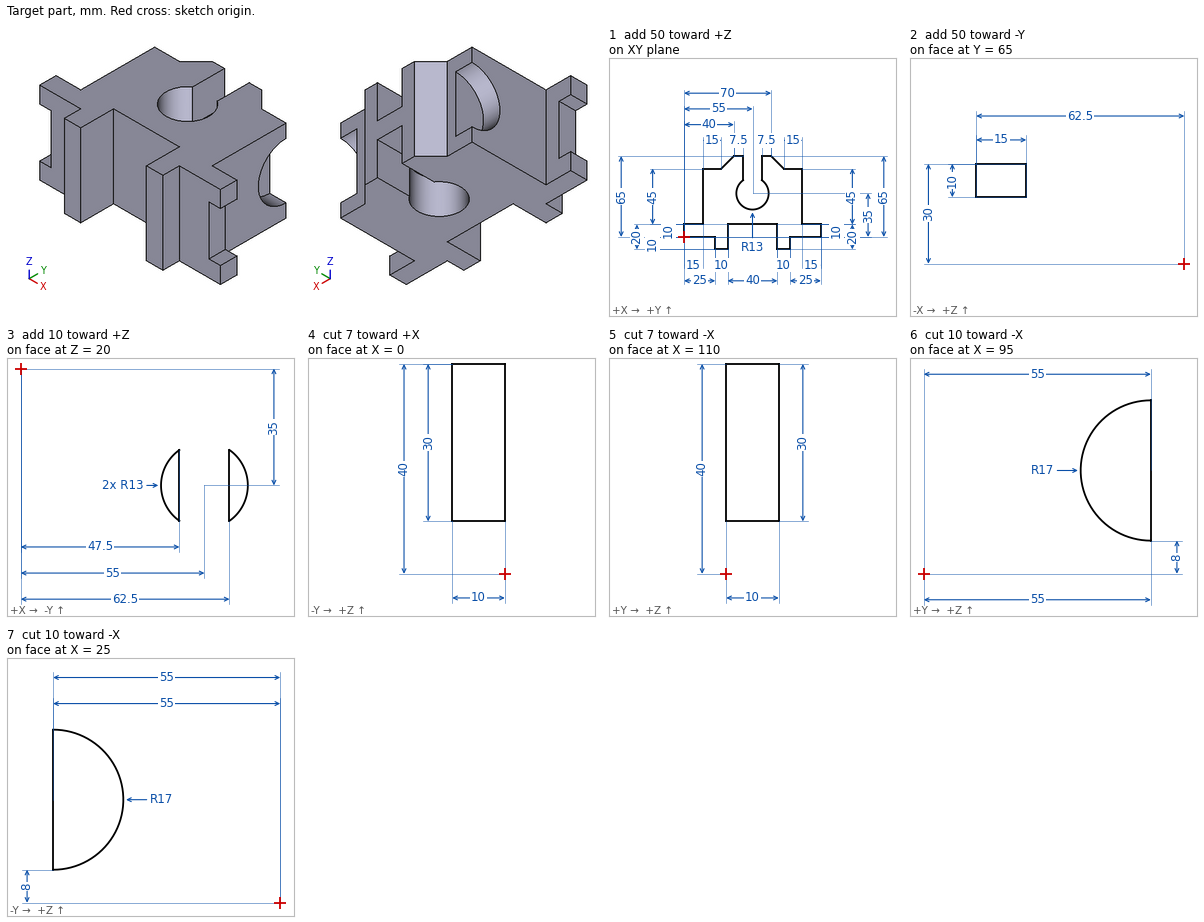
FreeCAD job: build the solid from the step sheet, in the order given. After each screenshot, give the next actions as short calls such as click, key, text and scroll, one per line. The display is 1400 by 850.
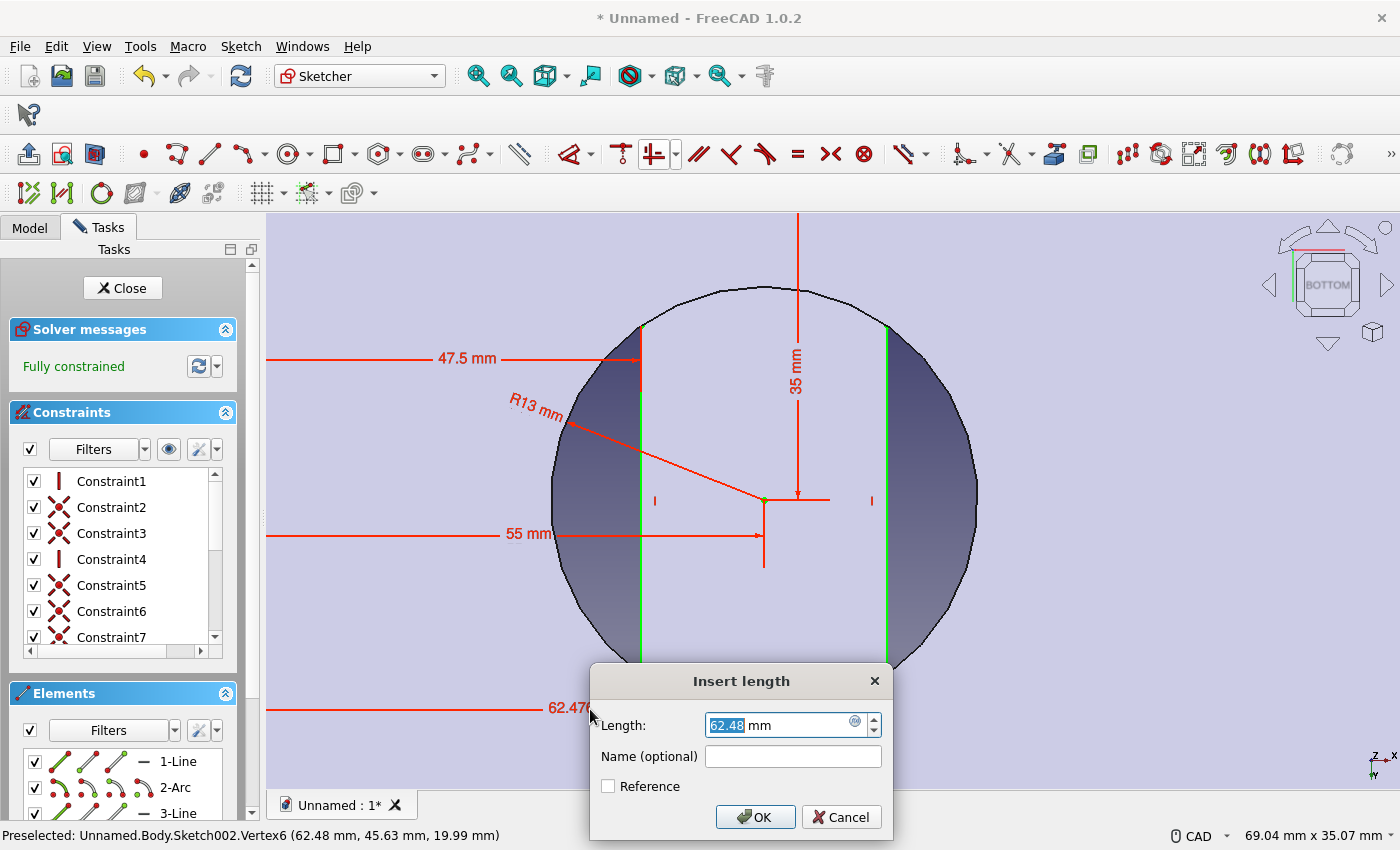
text(62.5)
key(Return)
key(Escape)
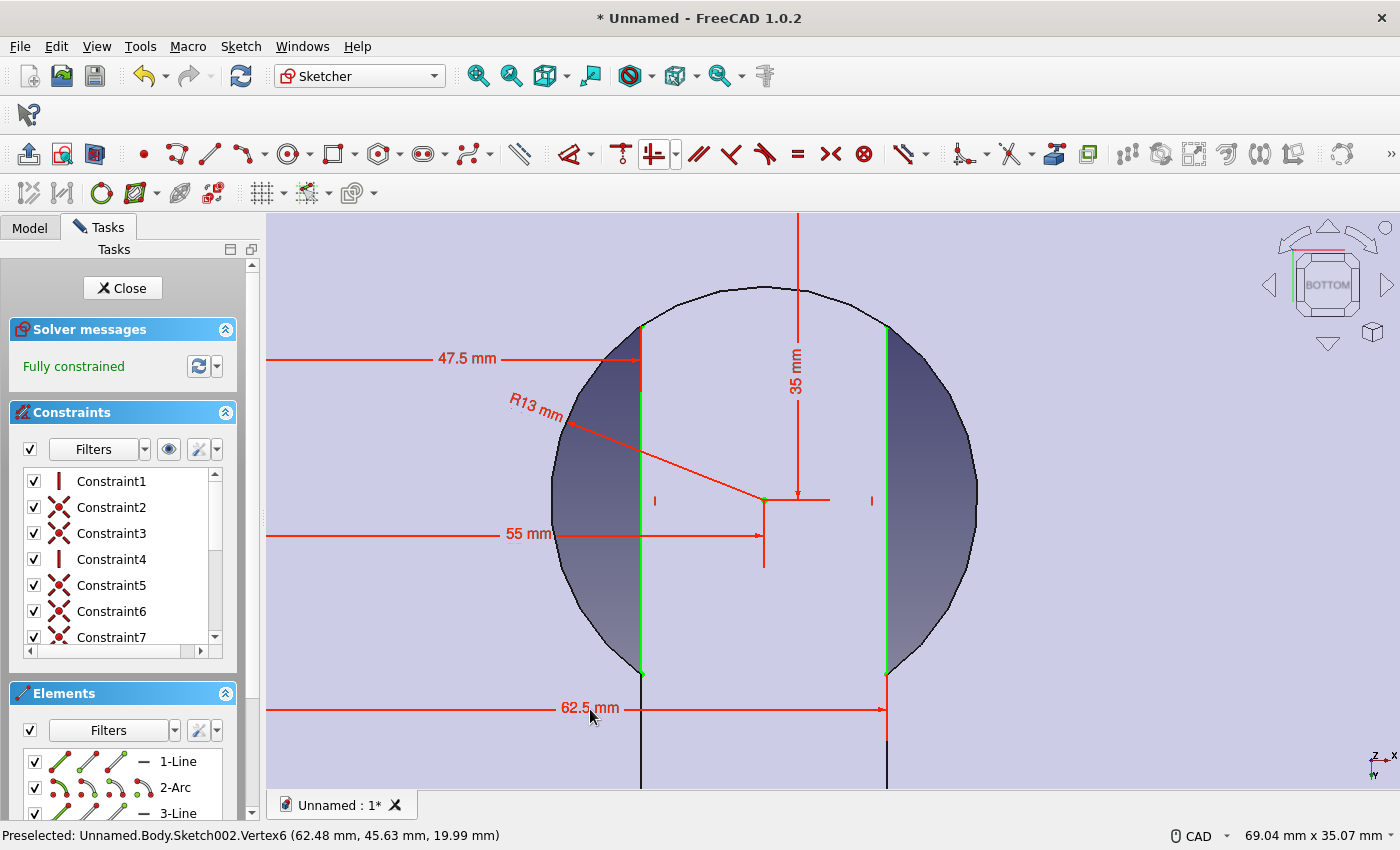
click(123, 288)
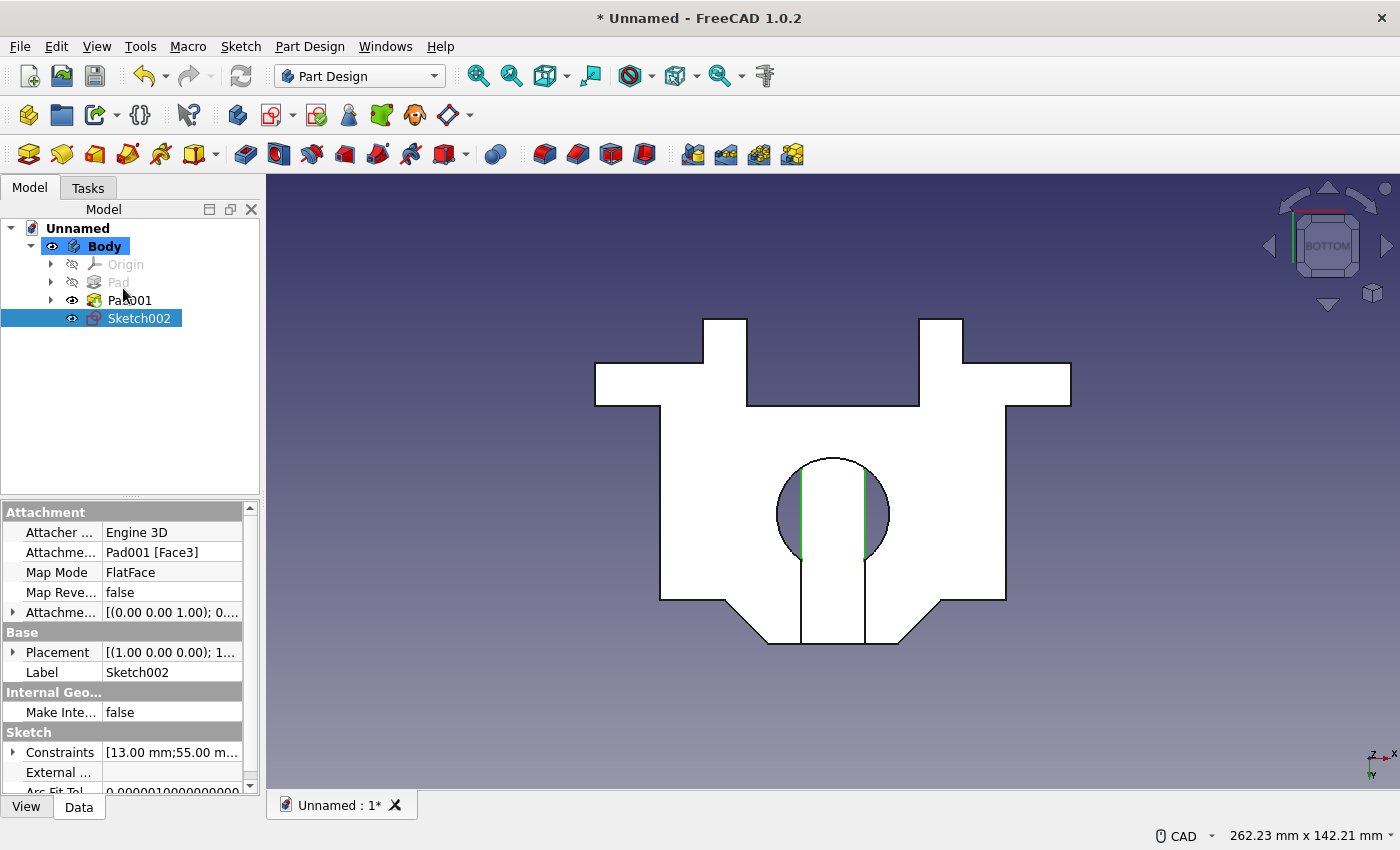
click(29, 154)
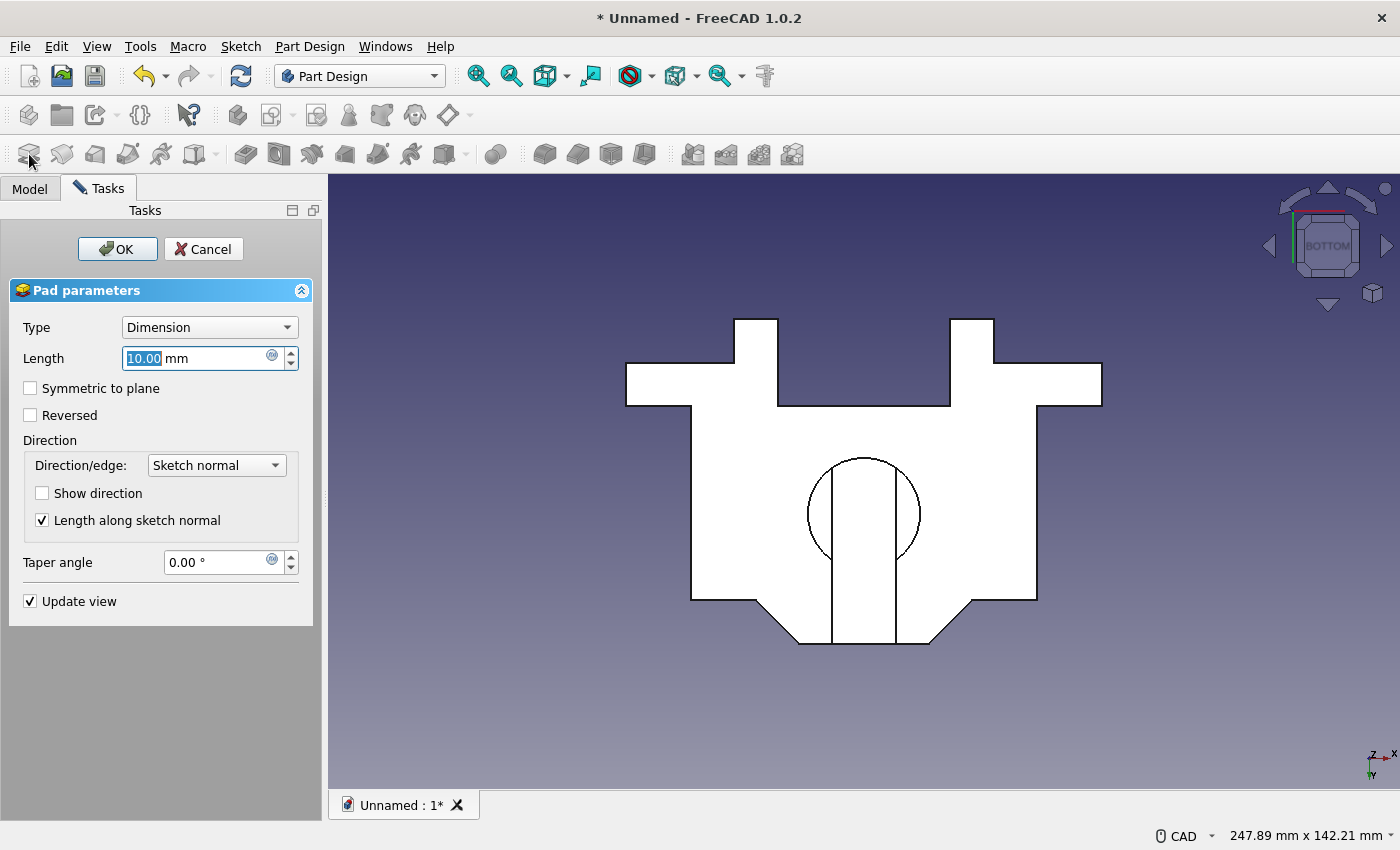
text(10)
key(Tab)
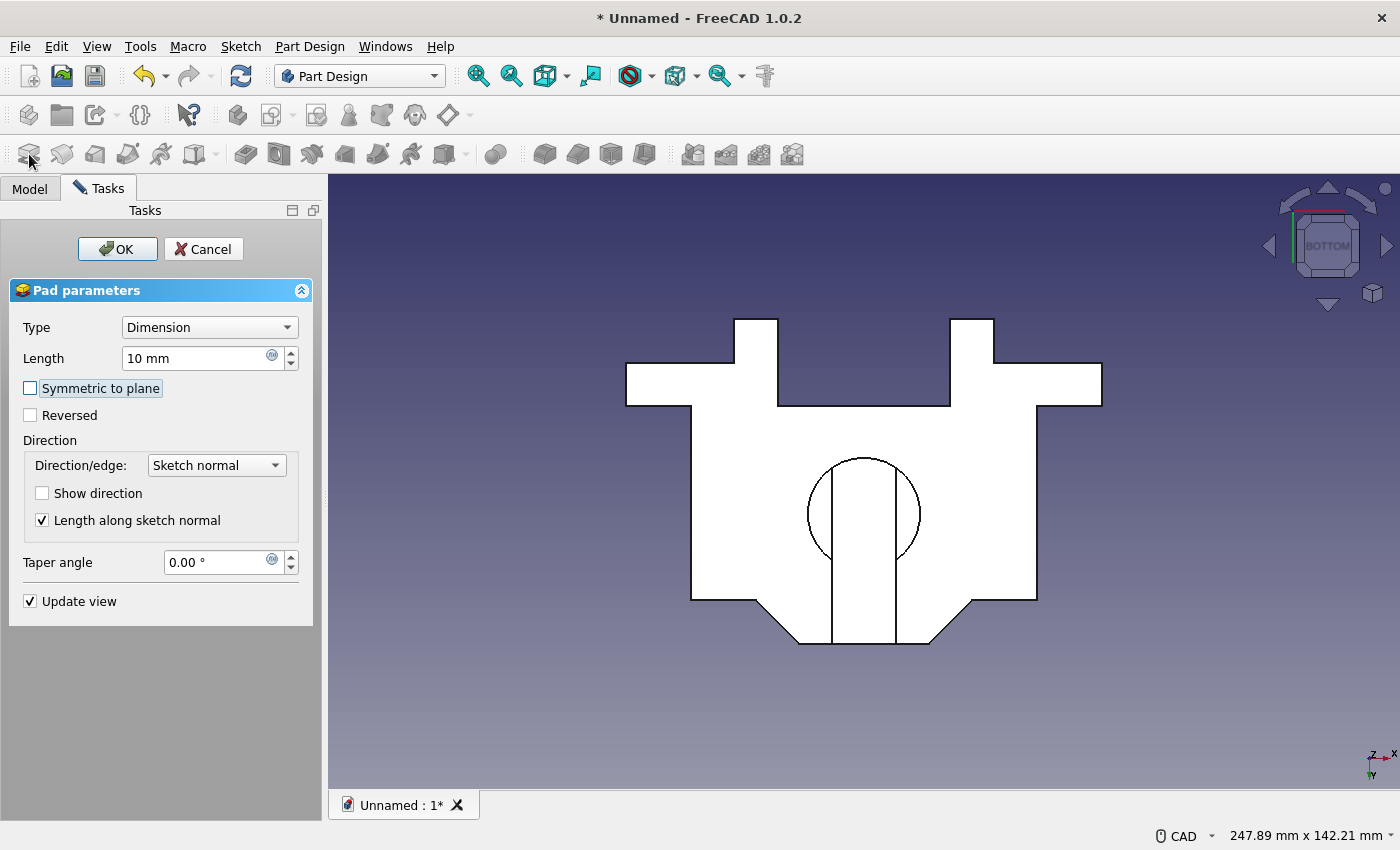
click(31, 415)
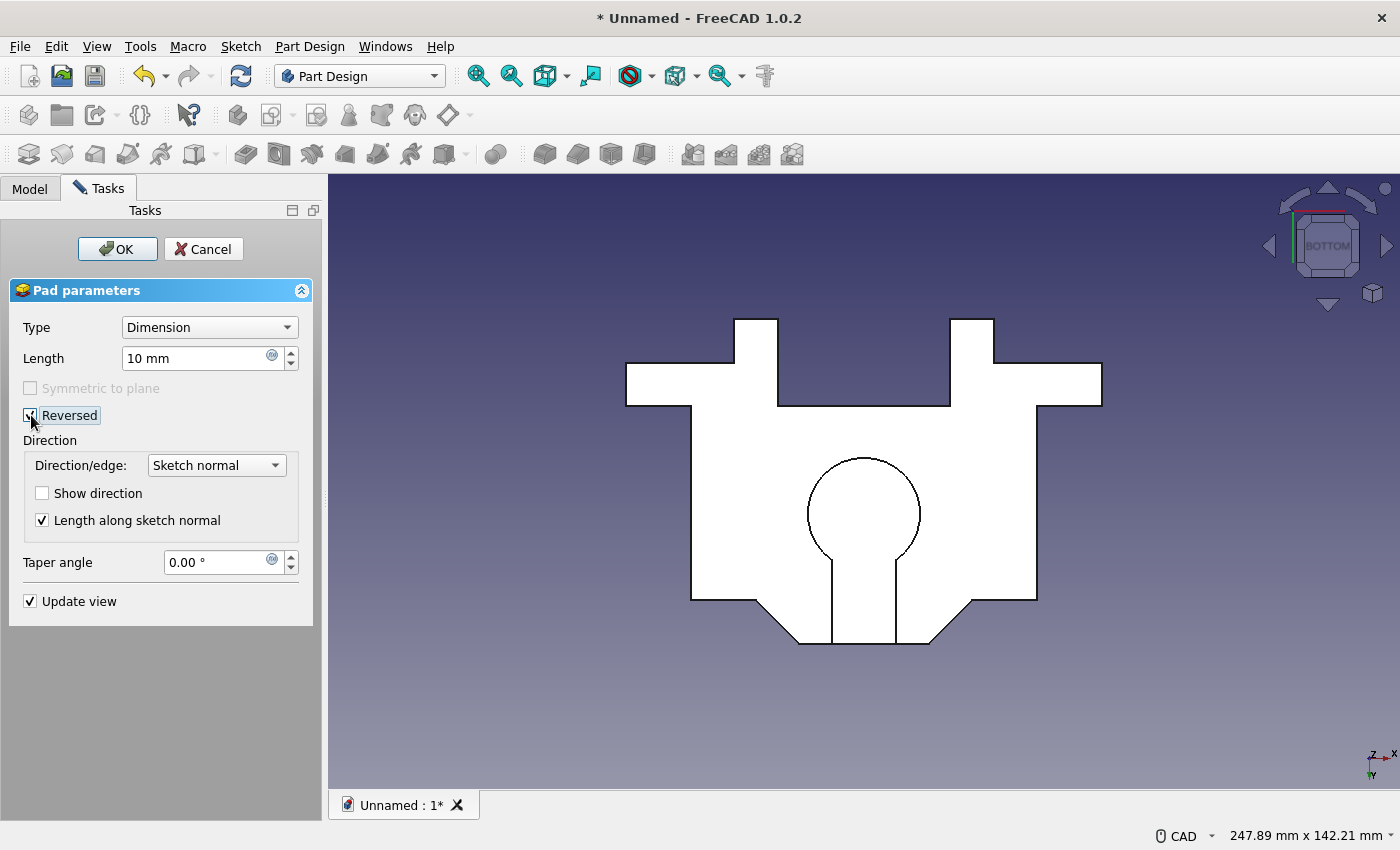
click(118, 249)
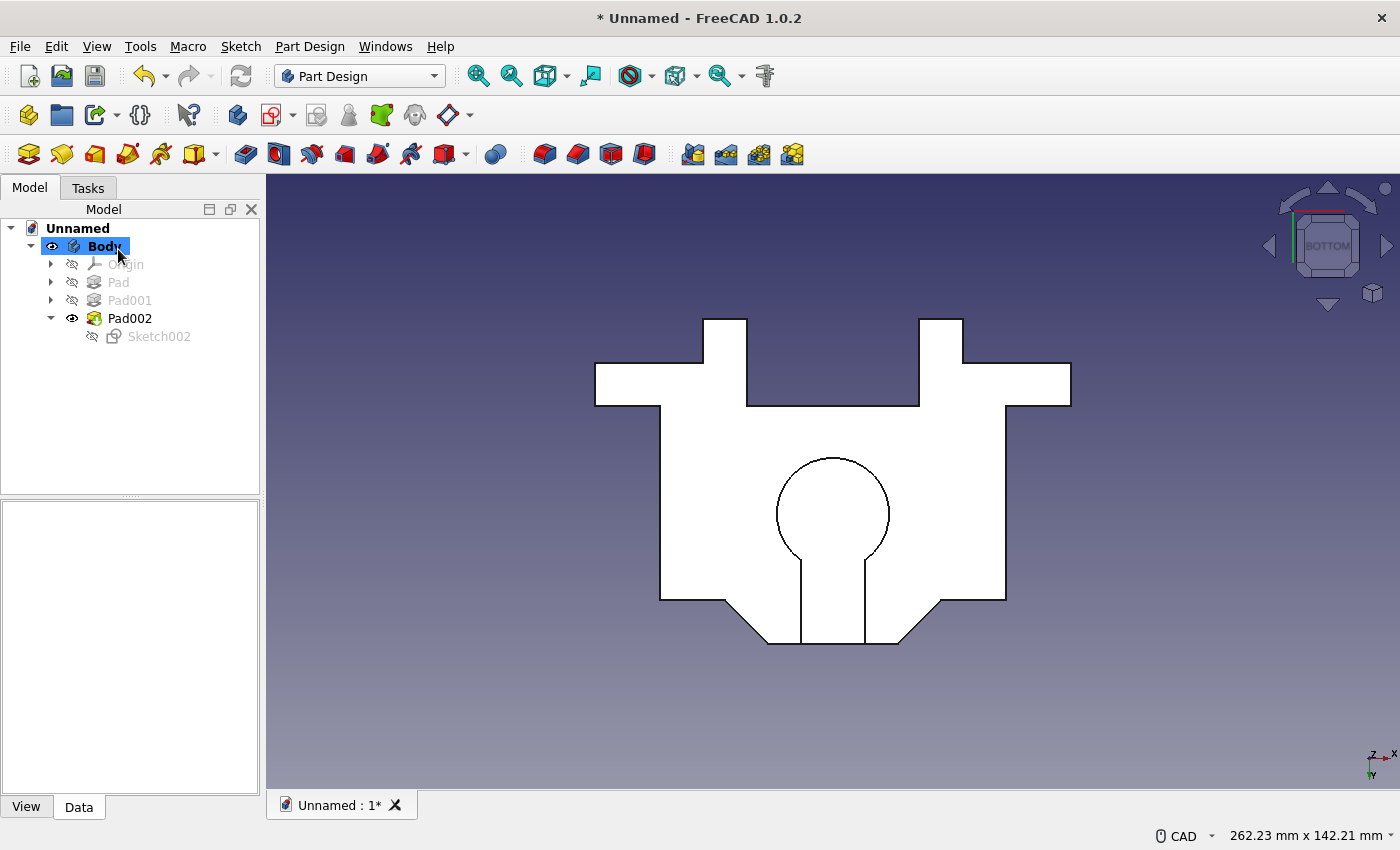
key(6)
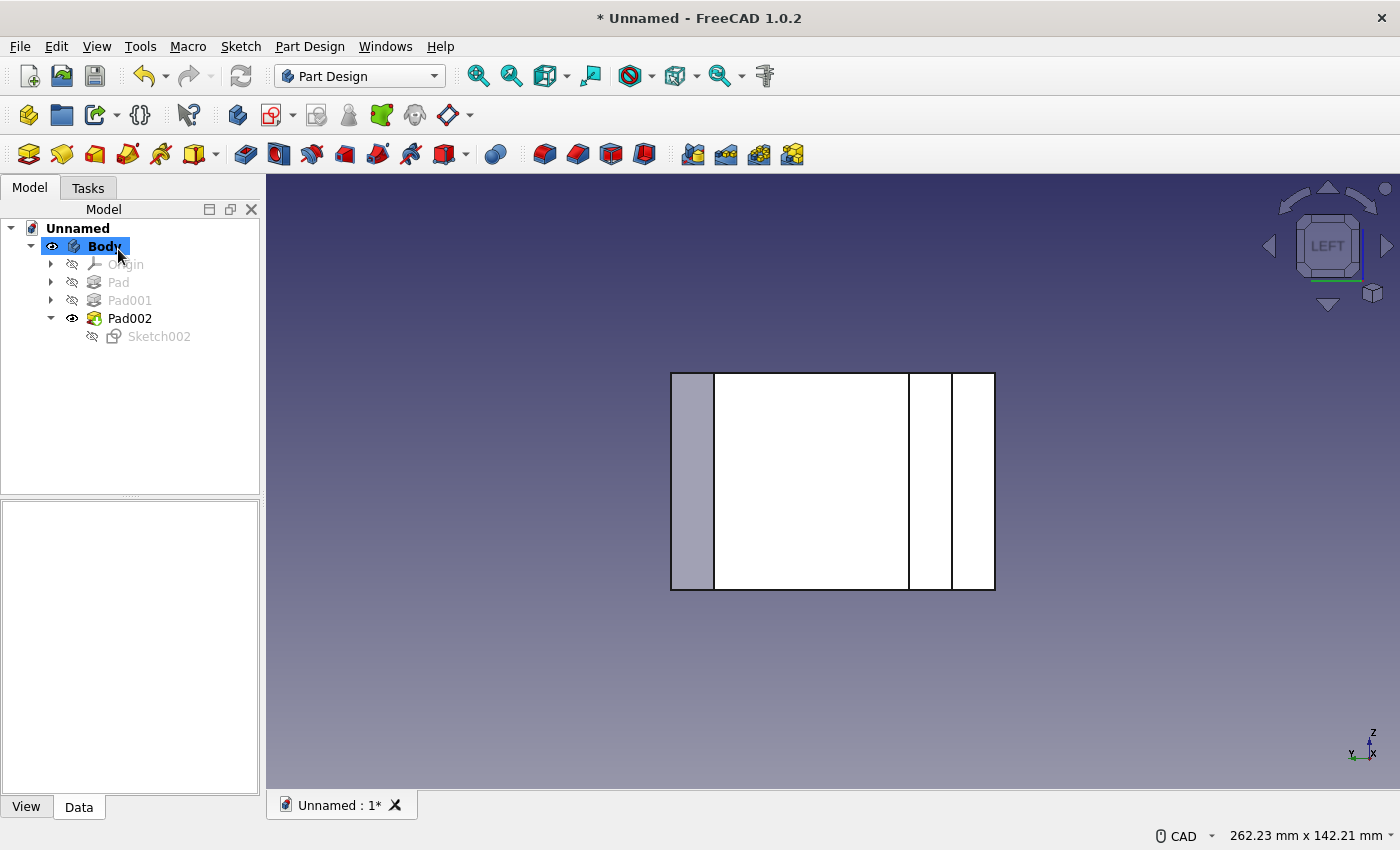
click(479, 76)